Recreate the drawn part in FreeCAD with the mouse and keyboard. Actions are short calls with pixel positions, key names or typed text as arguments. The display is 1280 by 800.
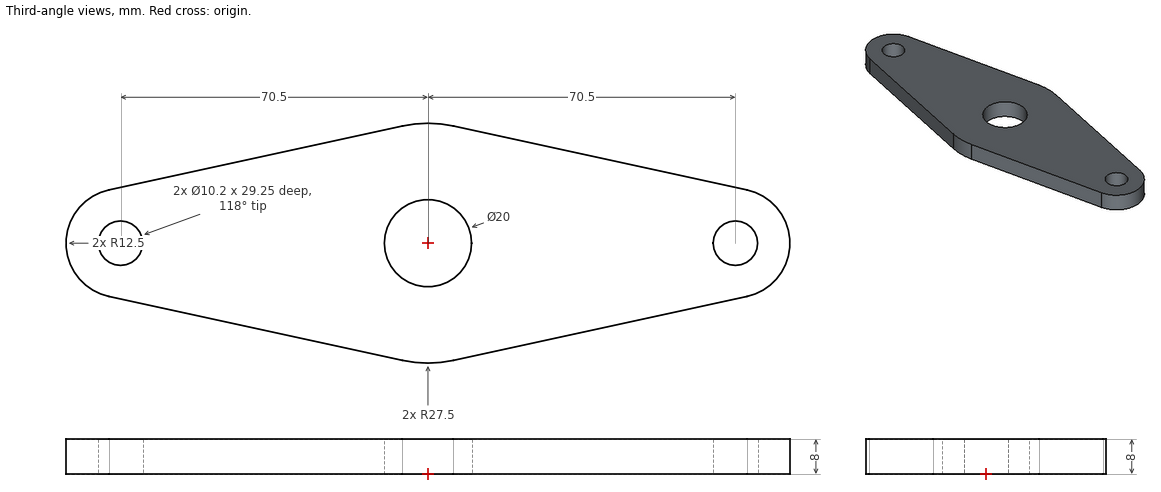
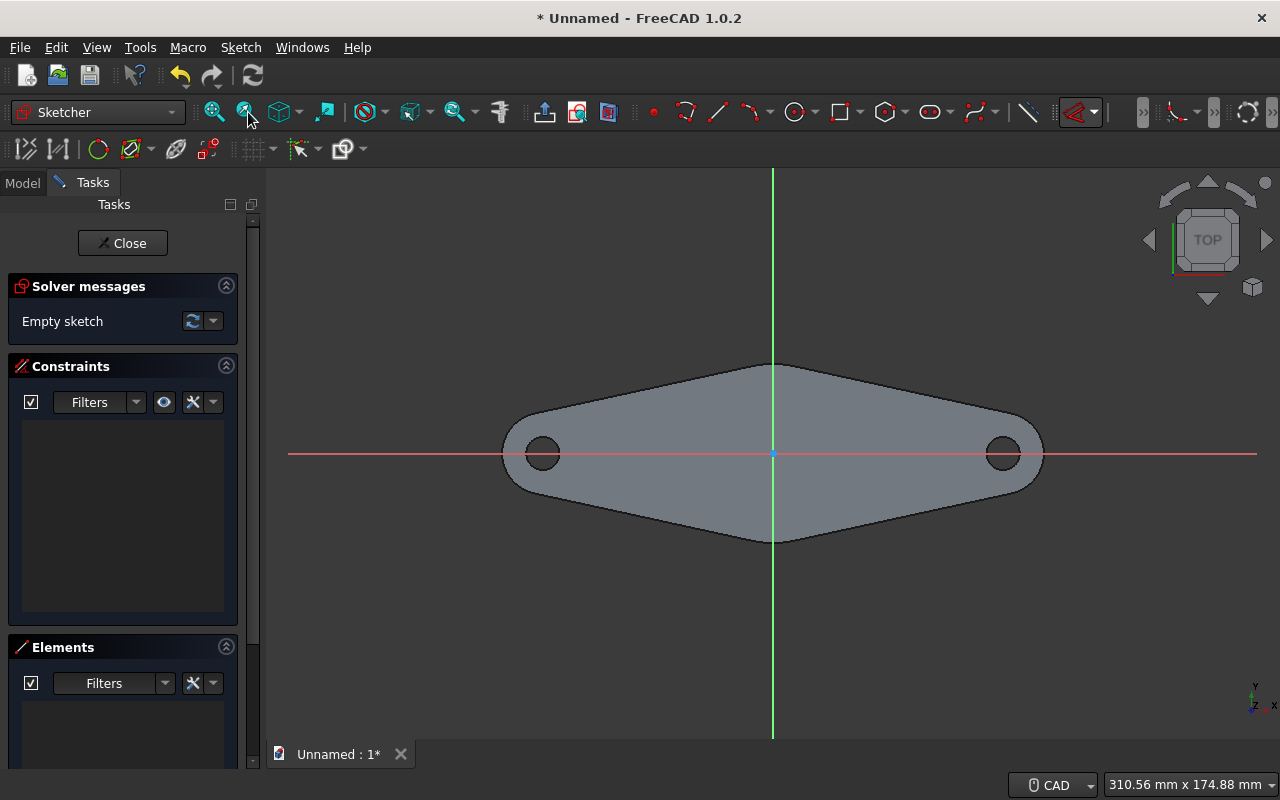
scroll(787, 454, up, 9)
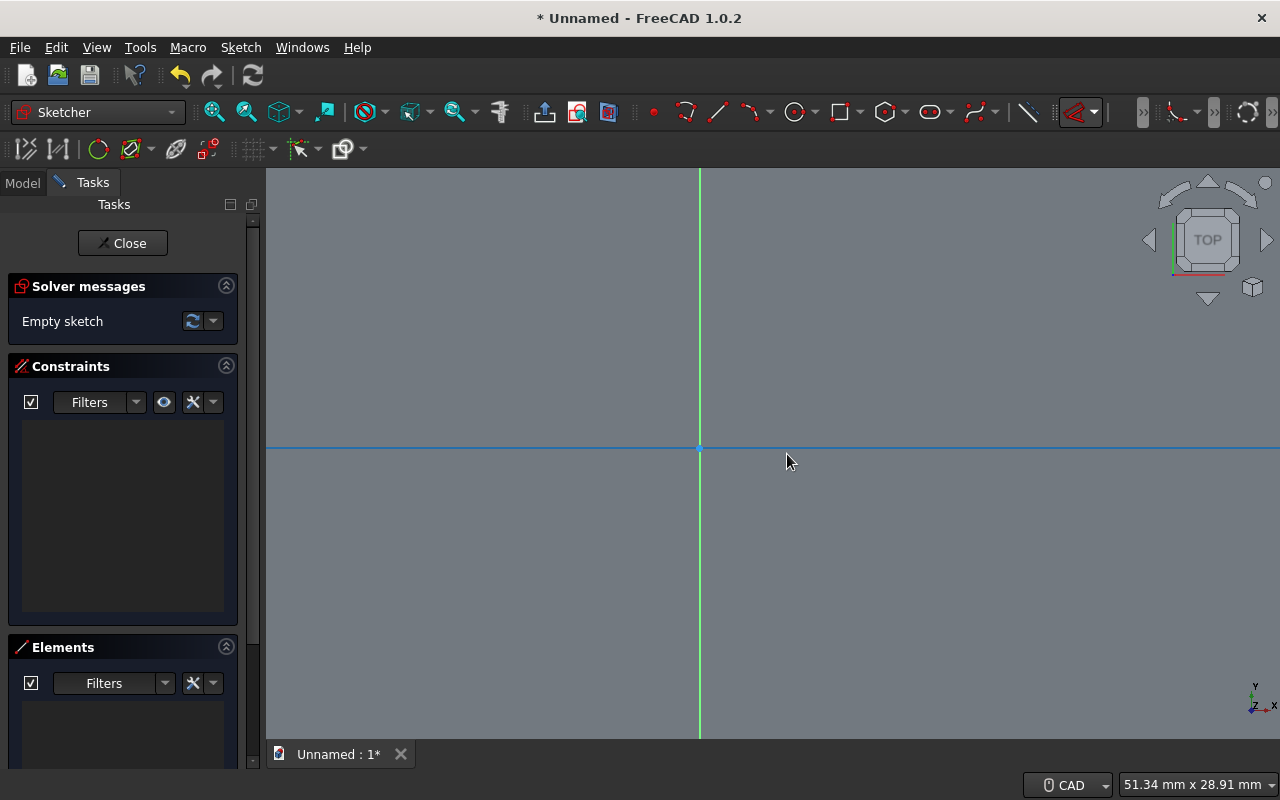
key(g)
key(c)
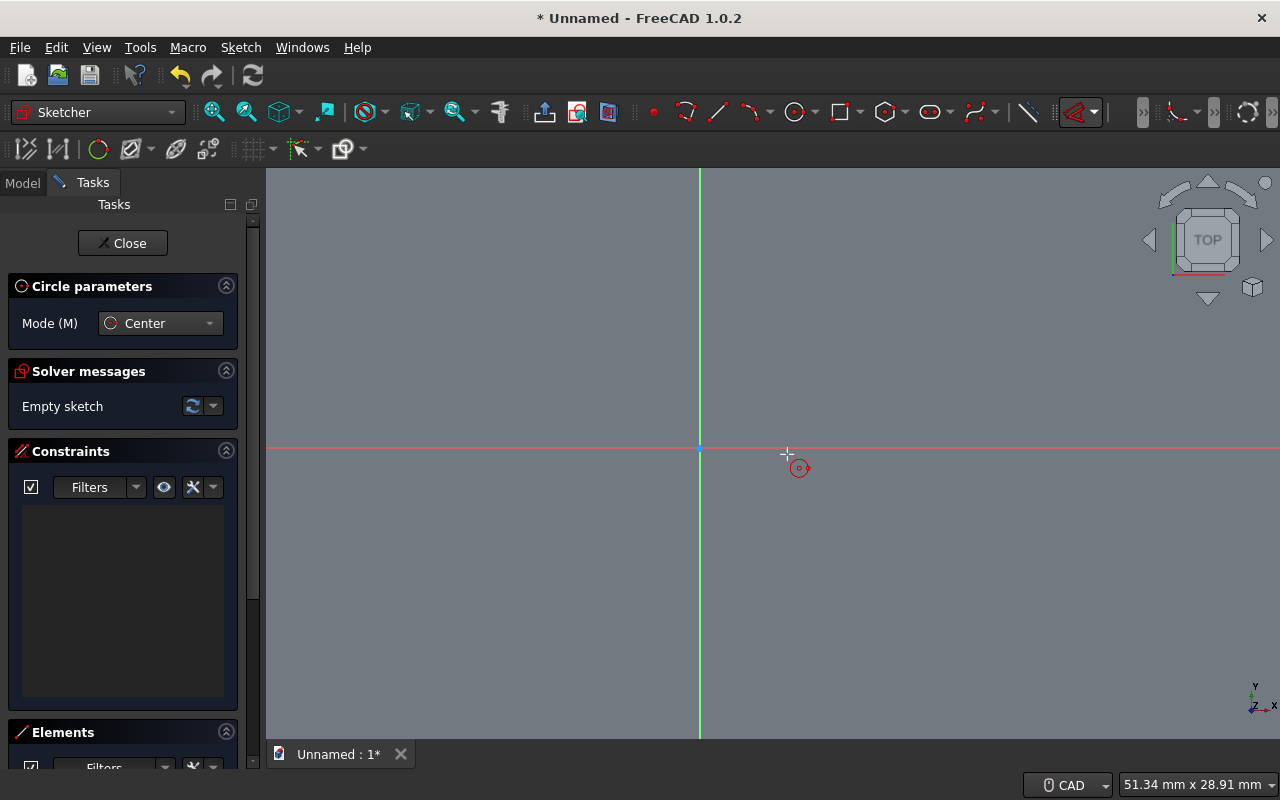
click(700, 448)
move(839, 309)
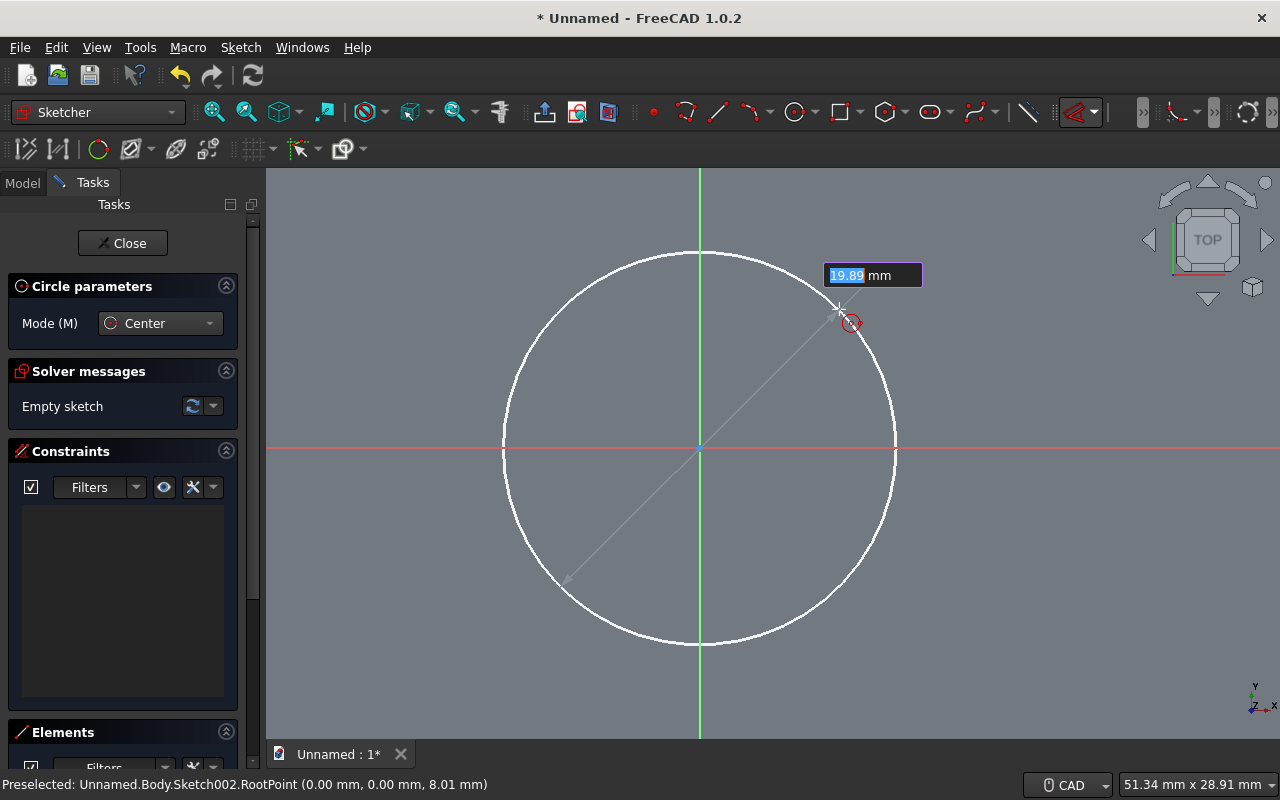
text(20)
key(Return)
key(Escape)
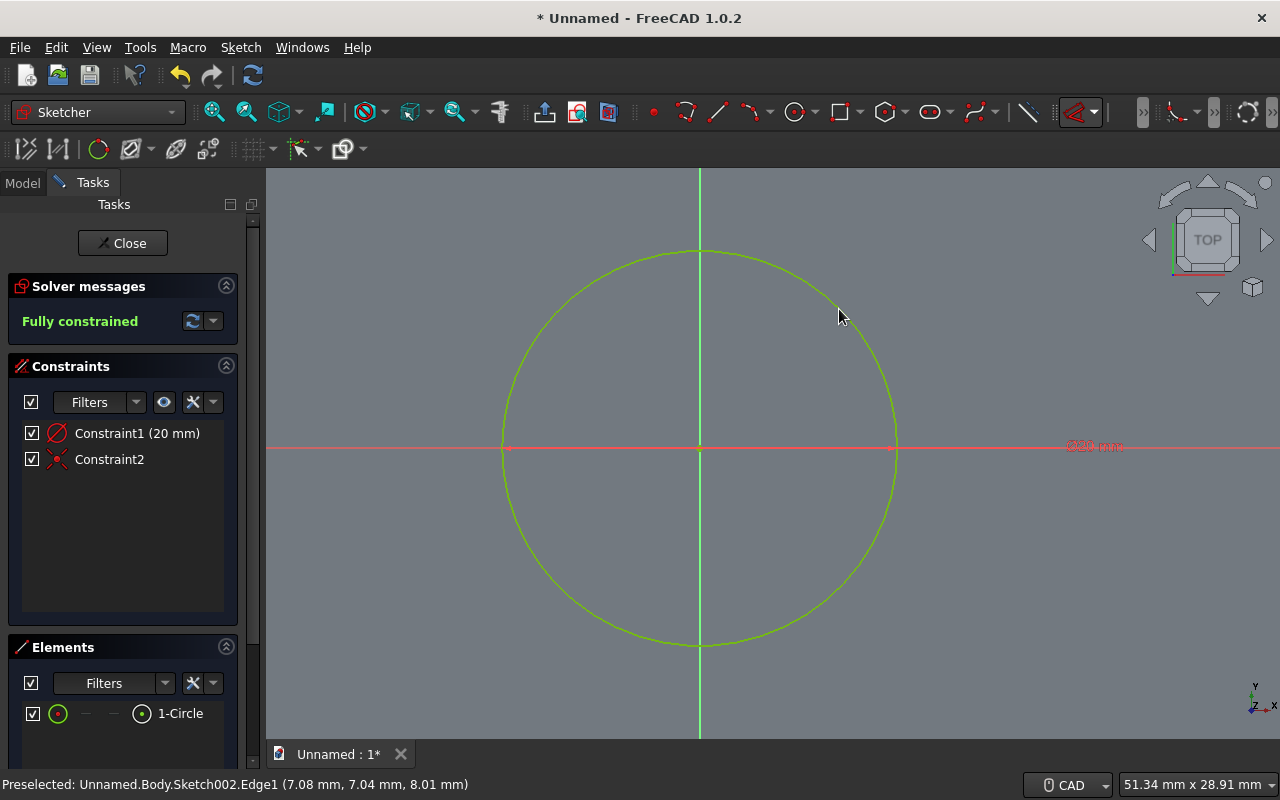
click(123, 243)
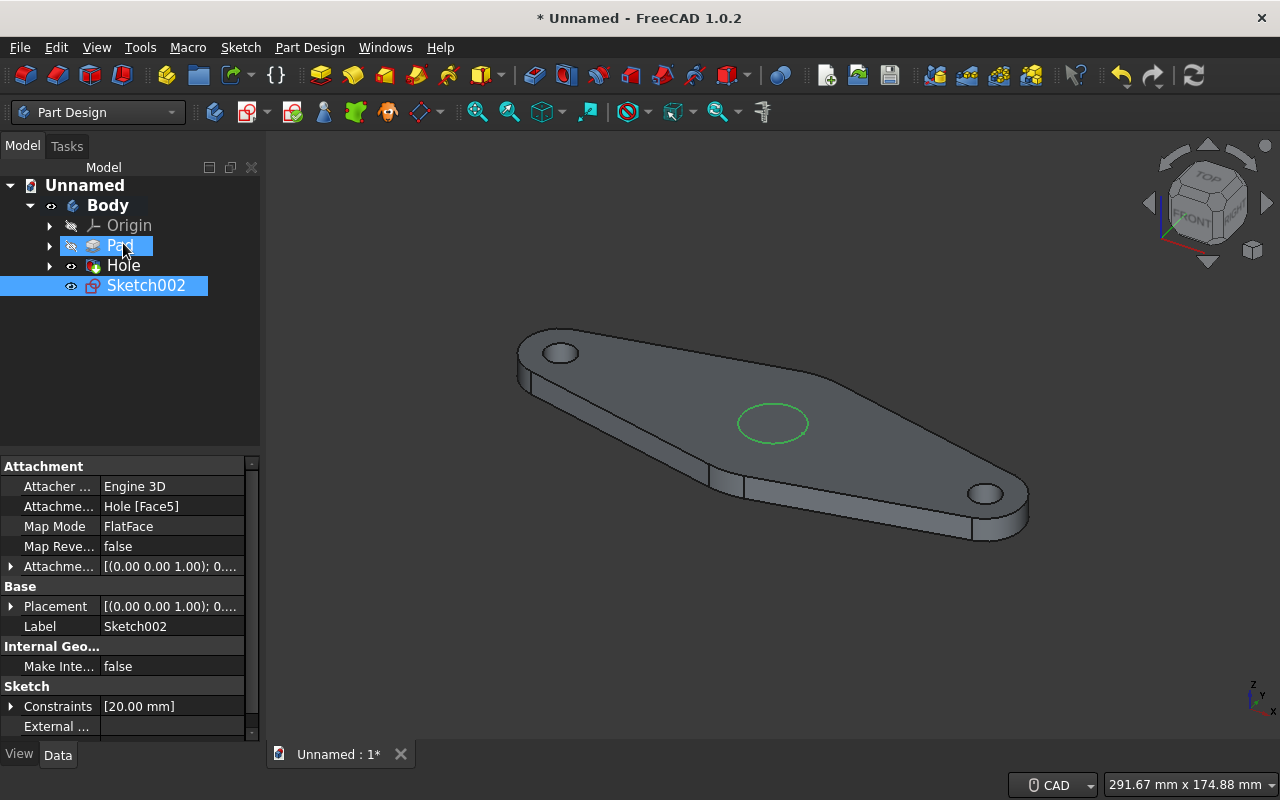
click(536, 76)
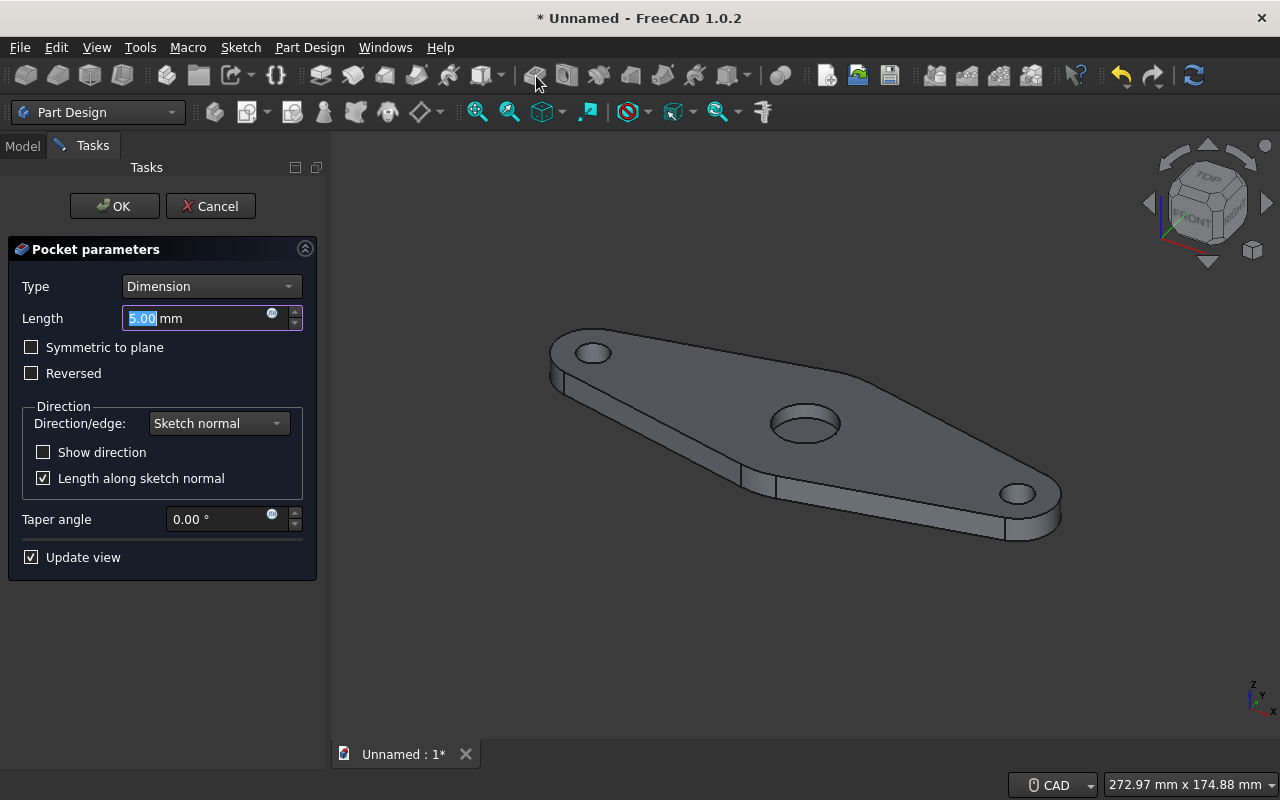
text(8)
key(Tab)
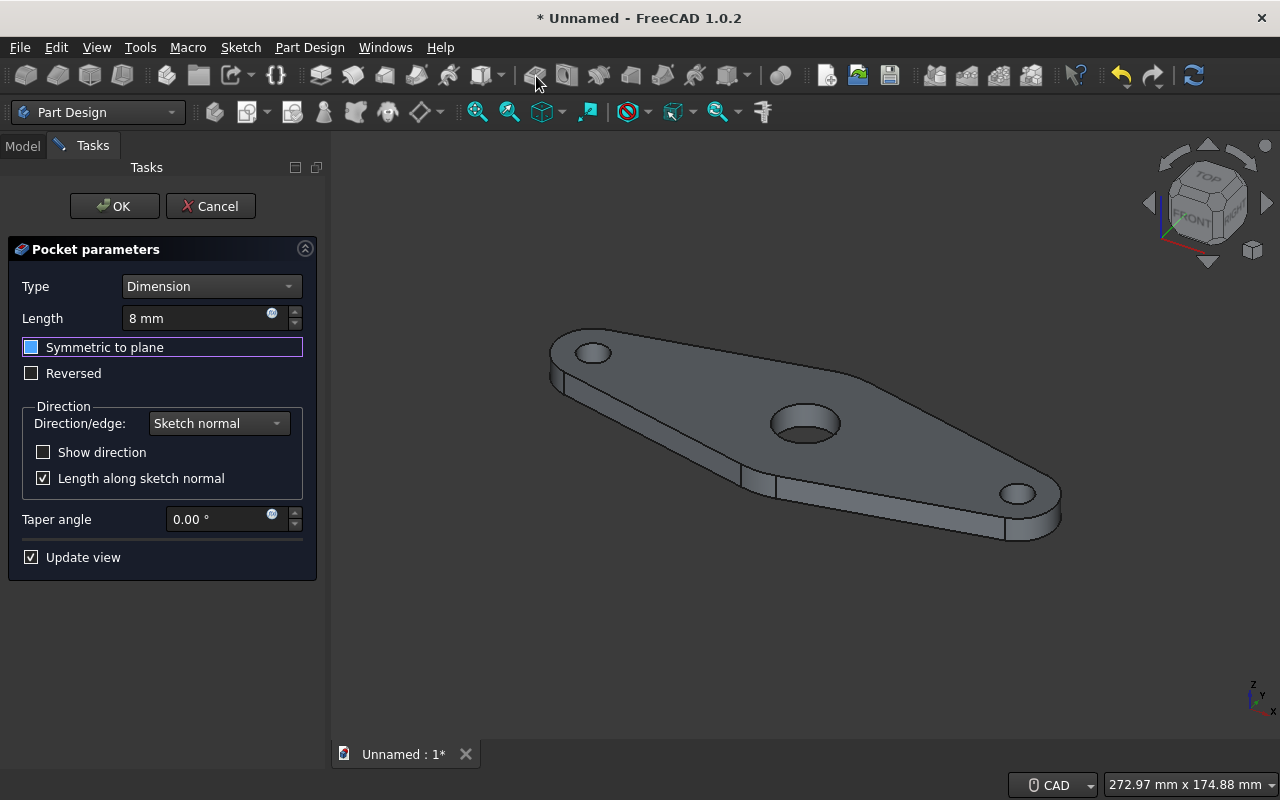
click(115, 206)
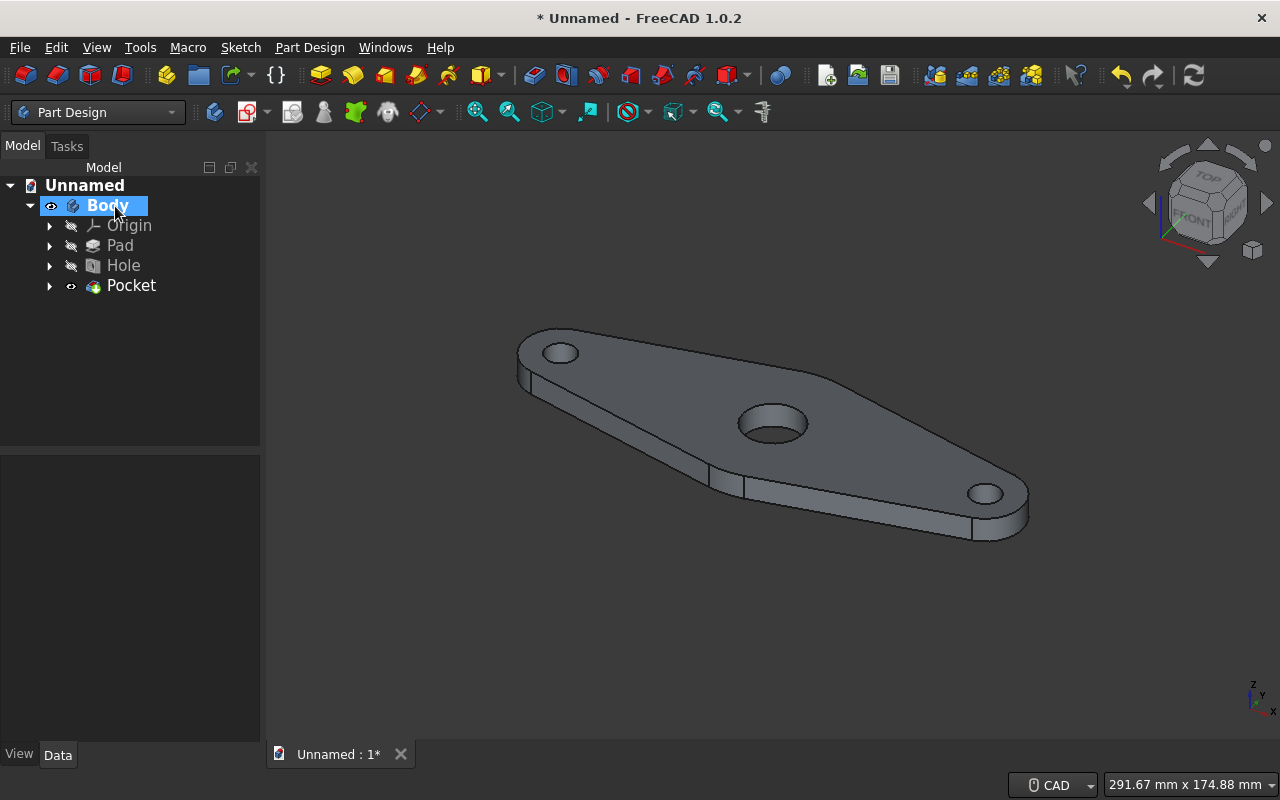
key(0)